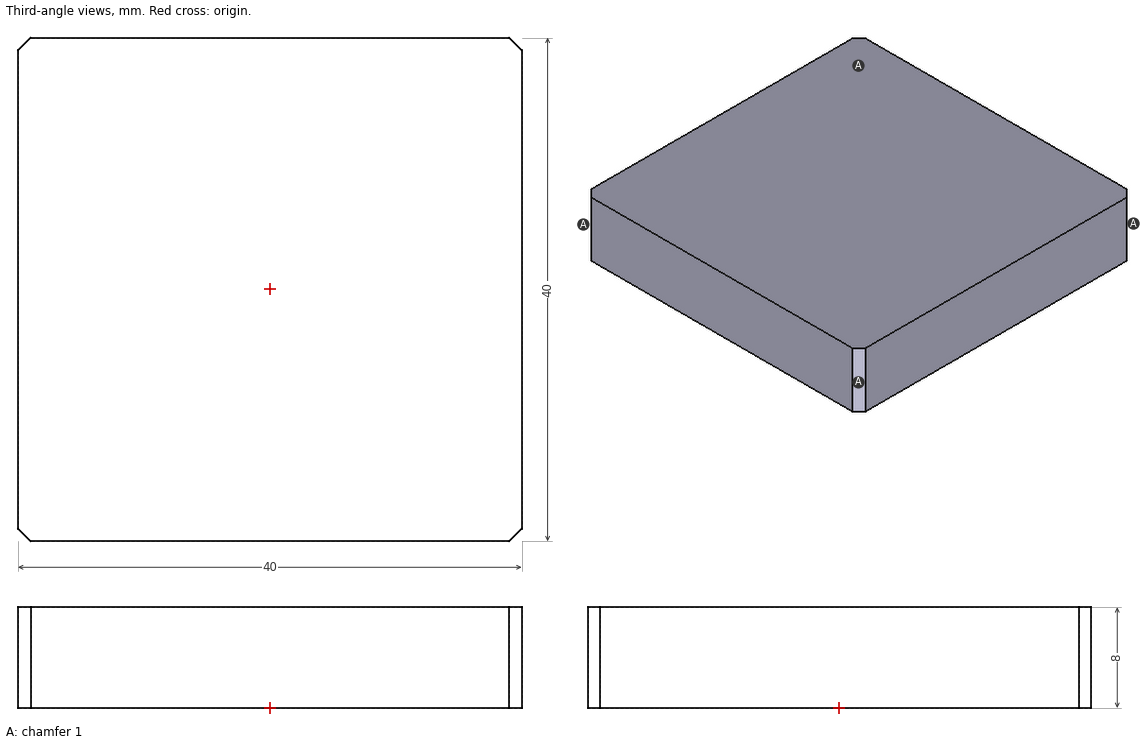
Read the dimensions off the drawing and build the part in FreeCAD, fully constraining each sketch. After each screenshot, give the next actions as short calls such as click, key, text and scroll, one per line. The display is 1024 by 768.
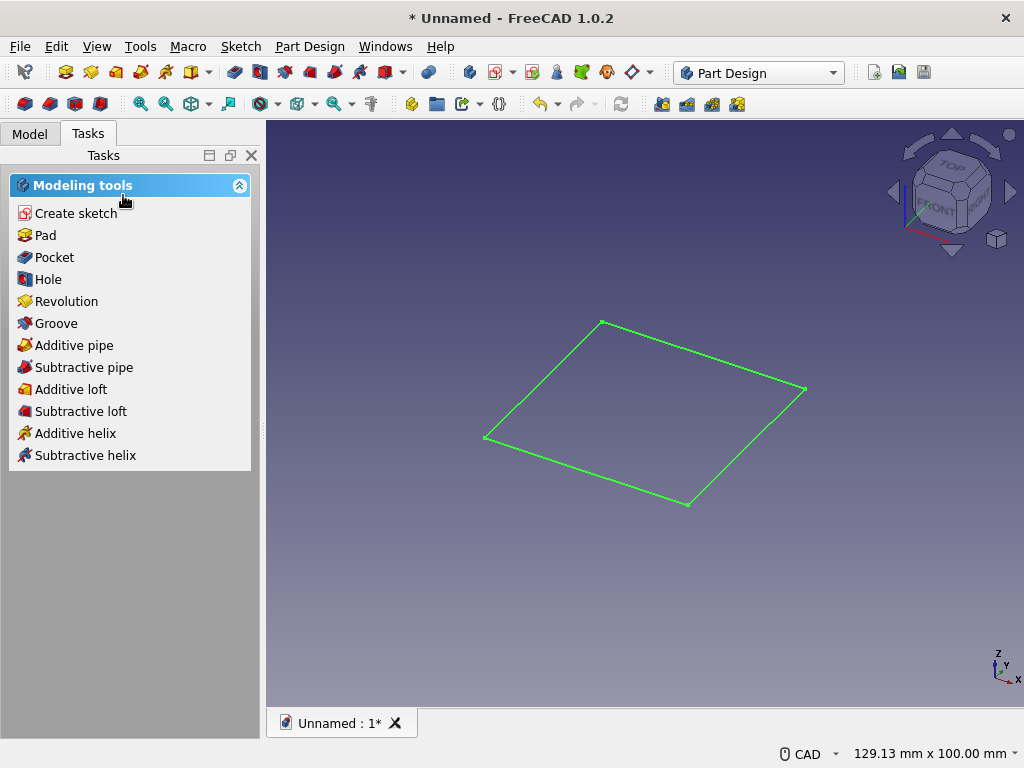
click(66, 72)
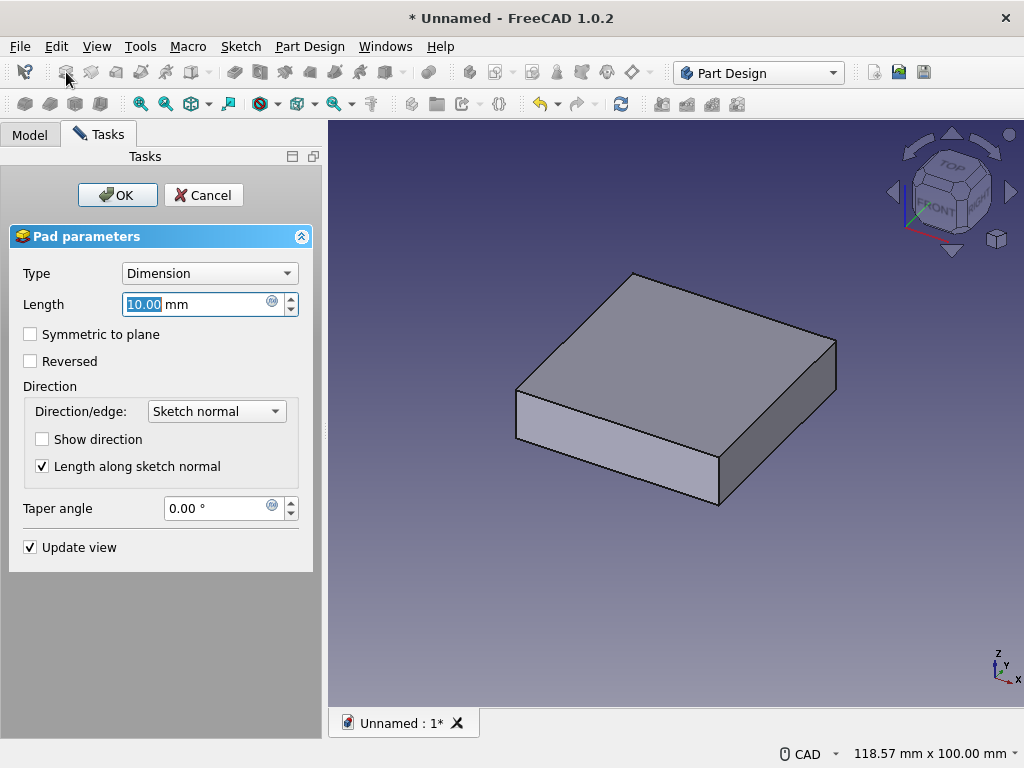
text(8)
key(Tab)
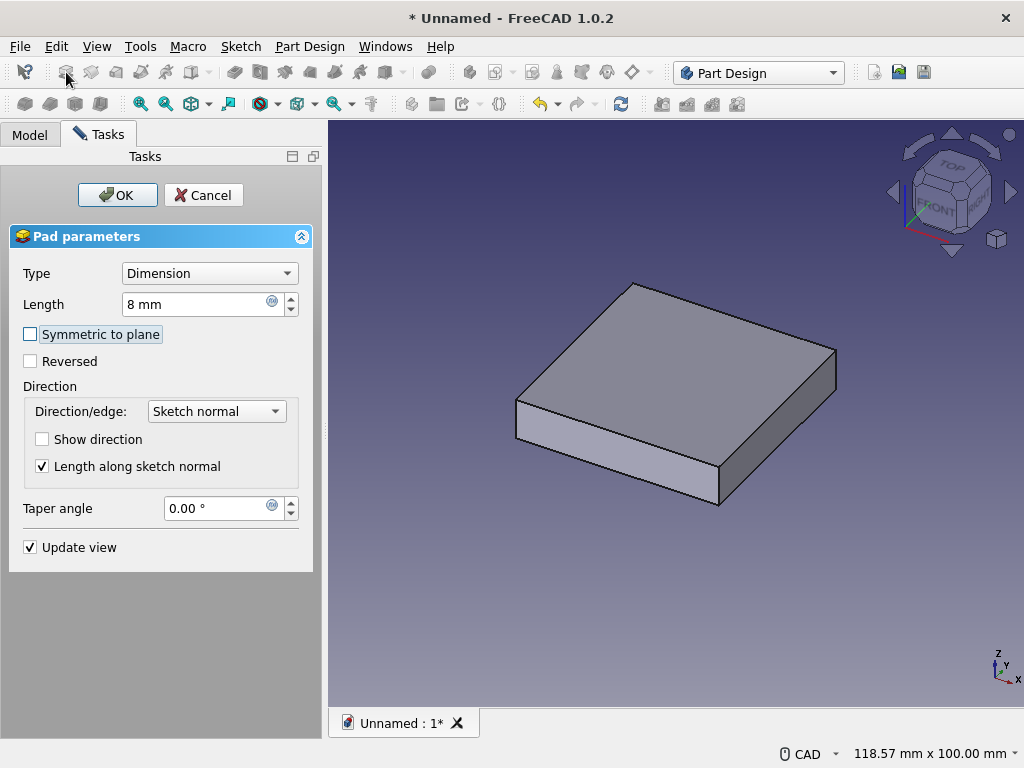
click(118, 195)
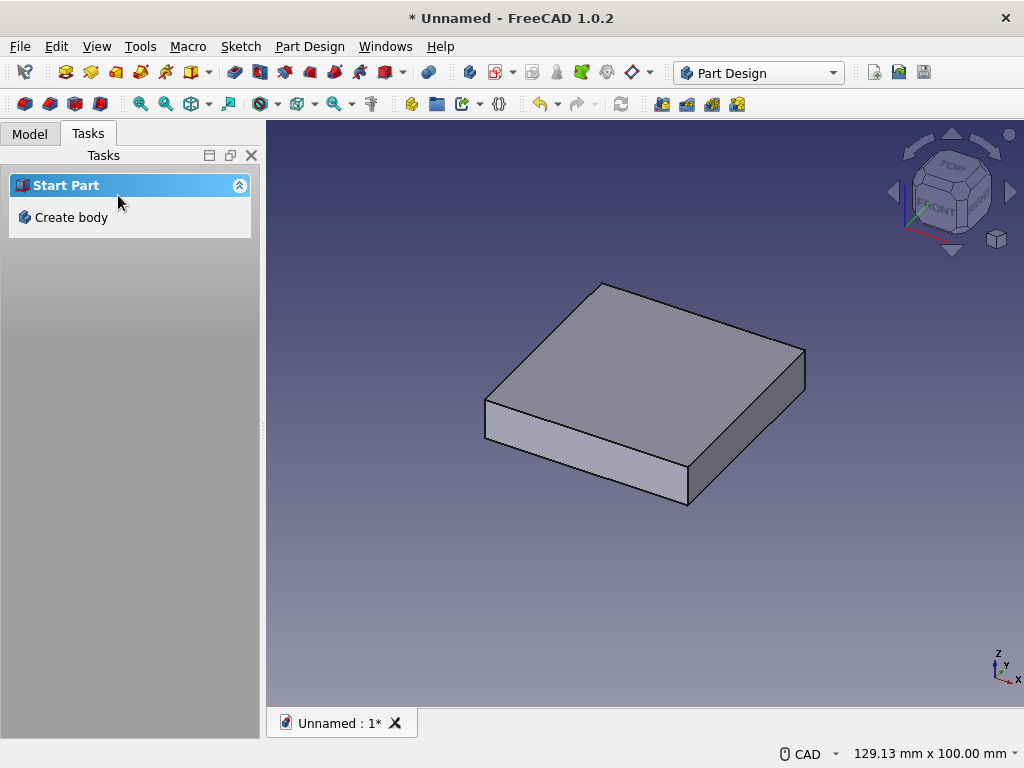
click(141, 104)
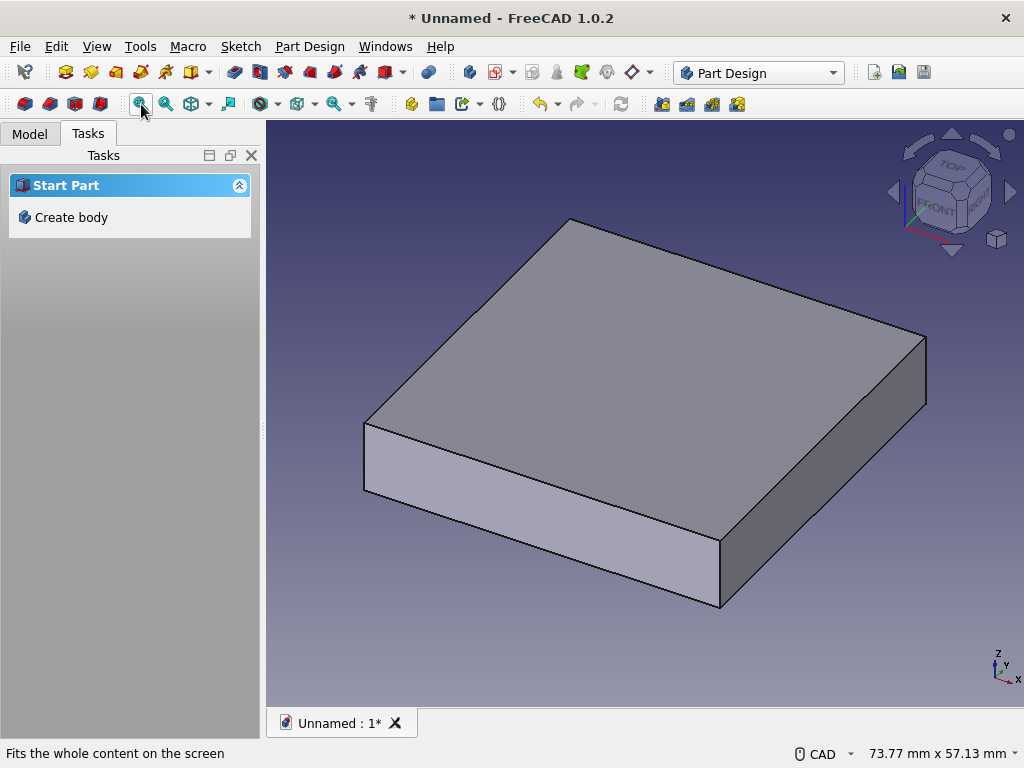
click(720, 574)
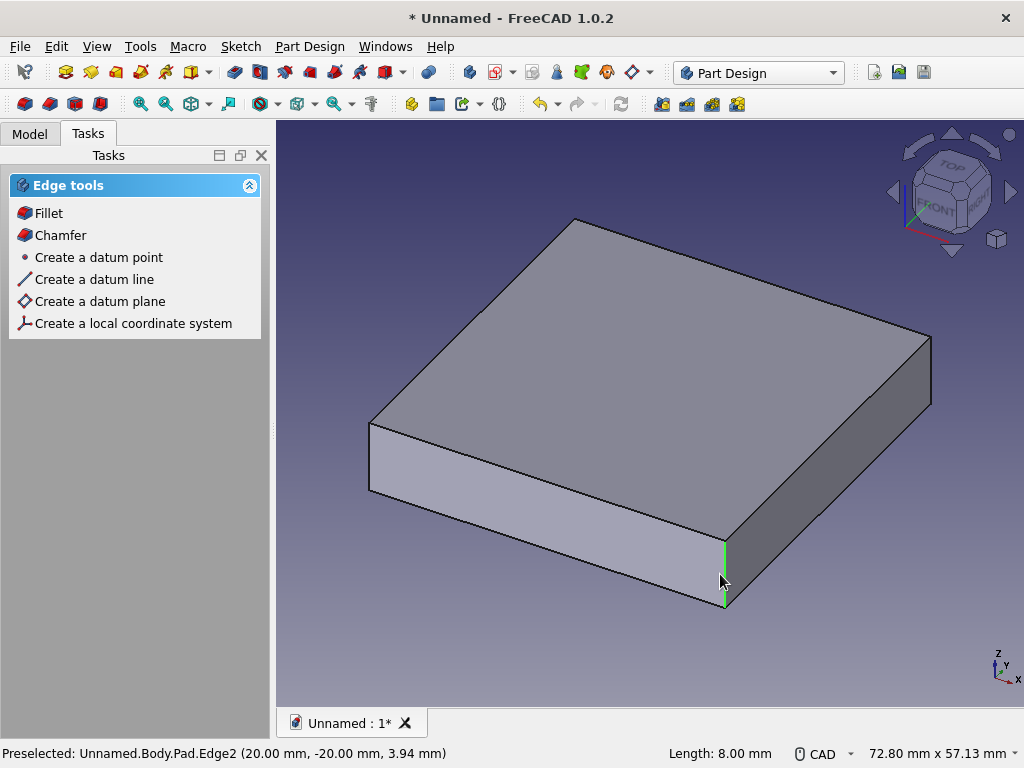
key(0)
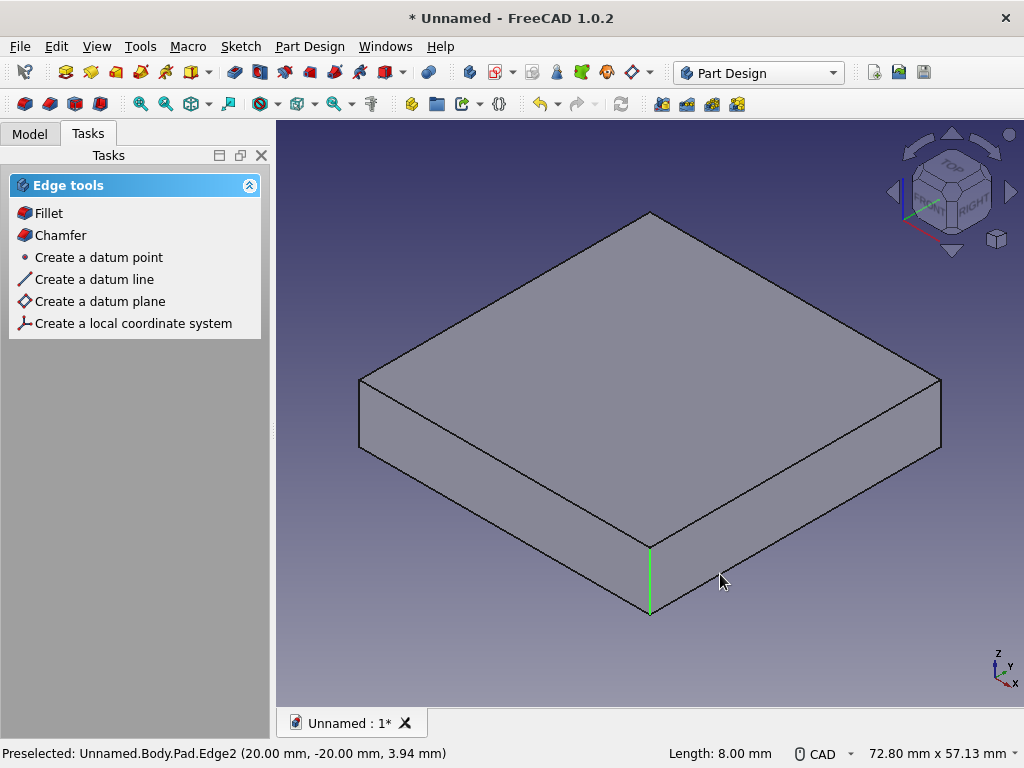
key(2)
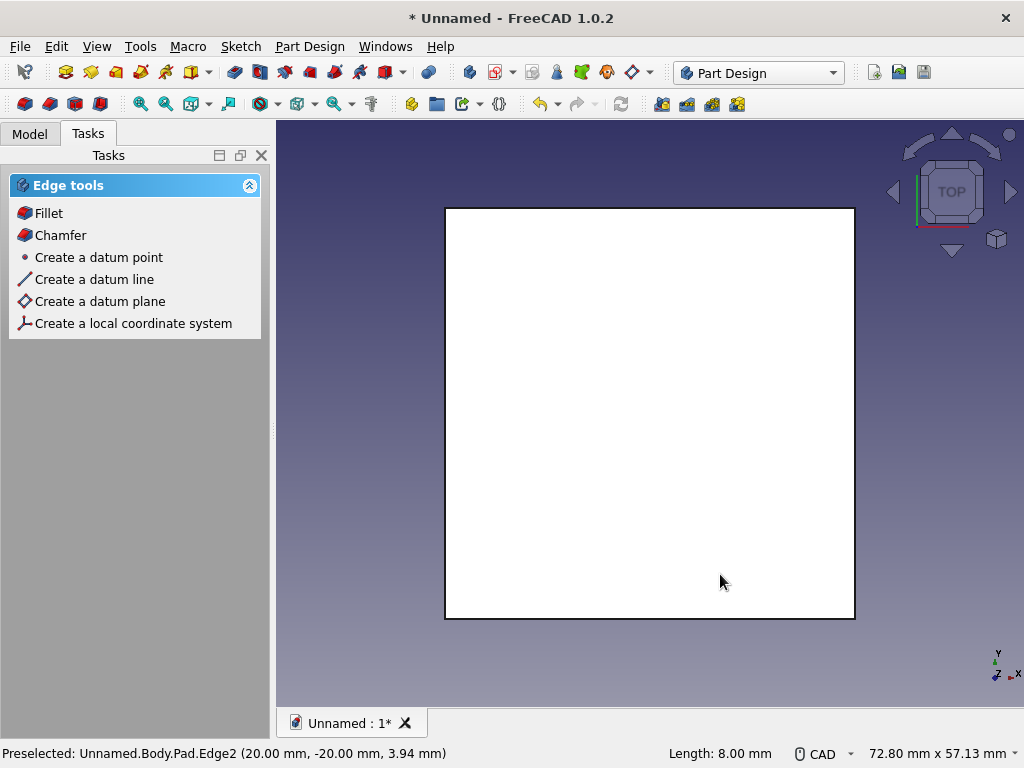
key(1)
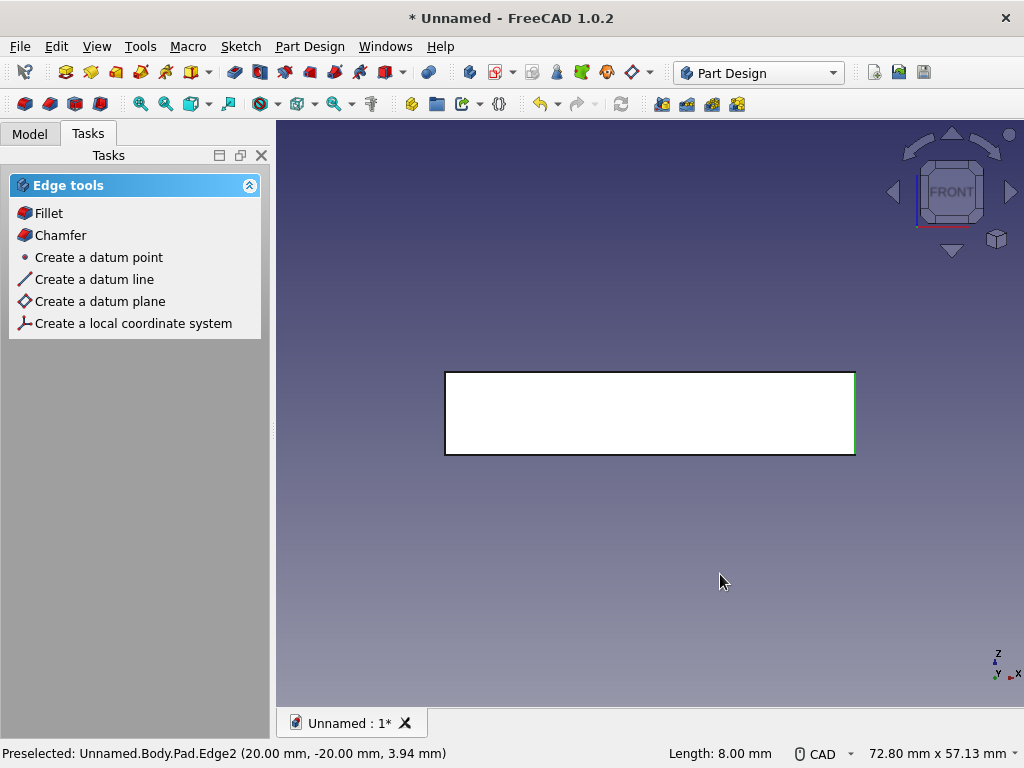
click(445, 412, ctrl)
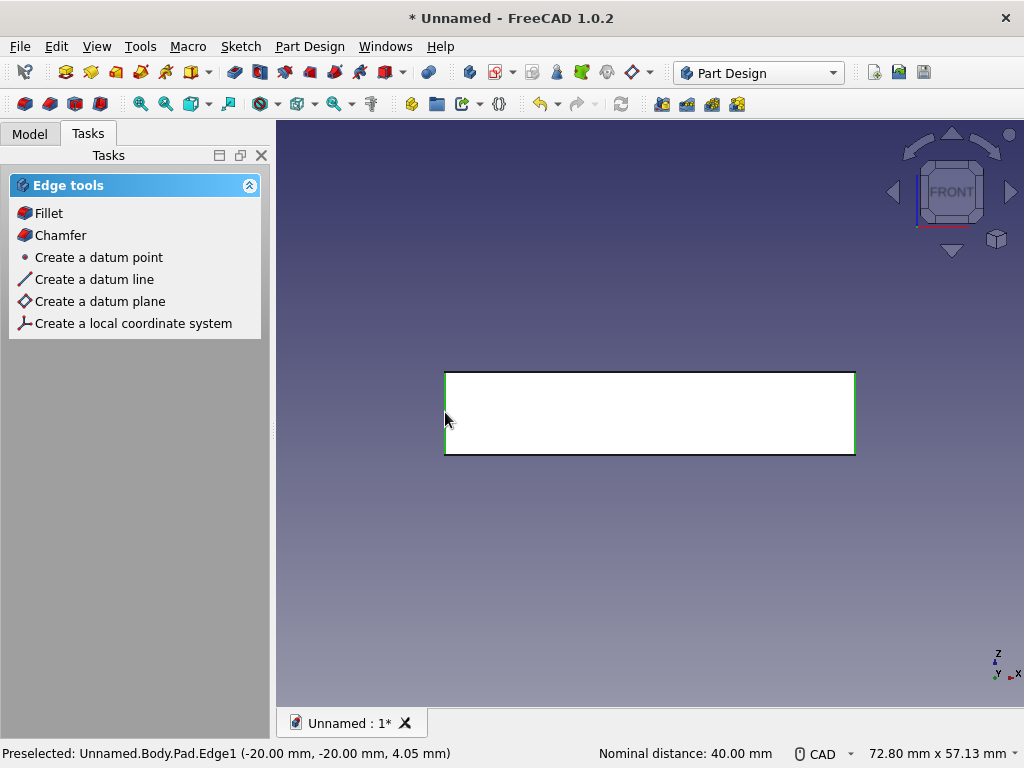
key(3)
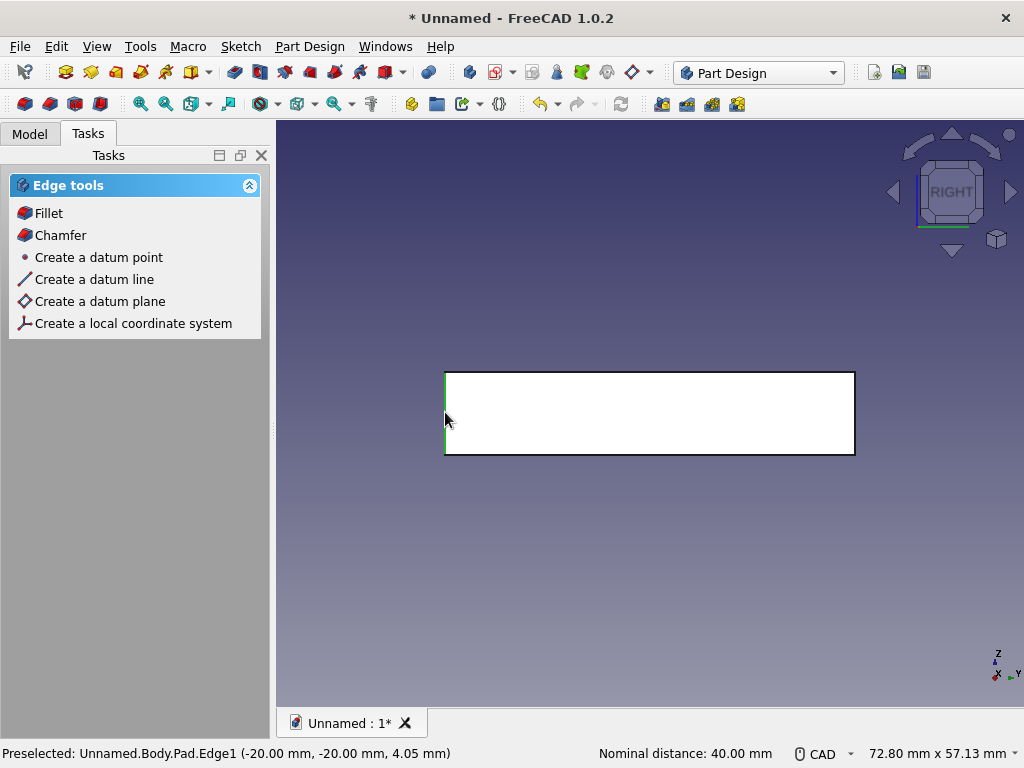
click(855, 412, ctrl)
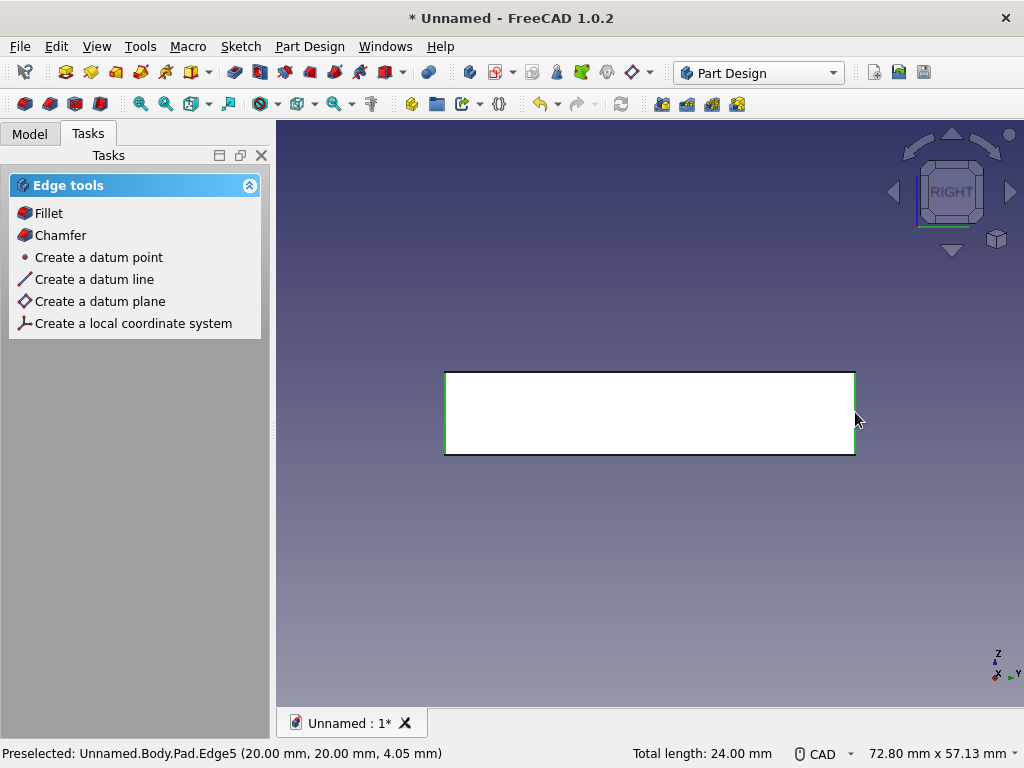
key(5)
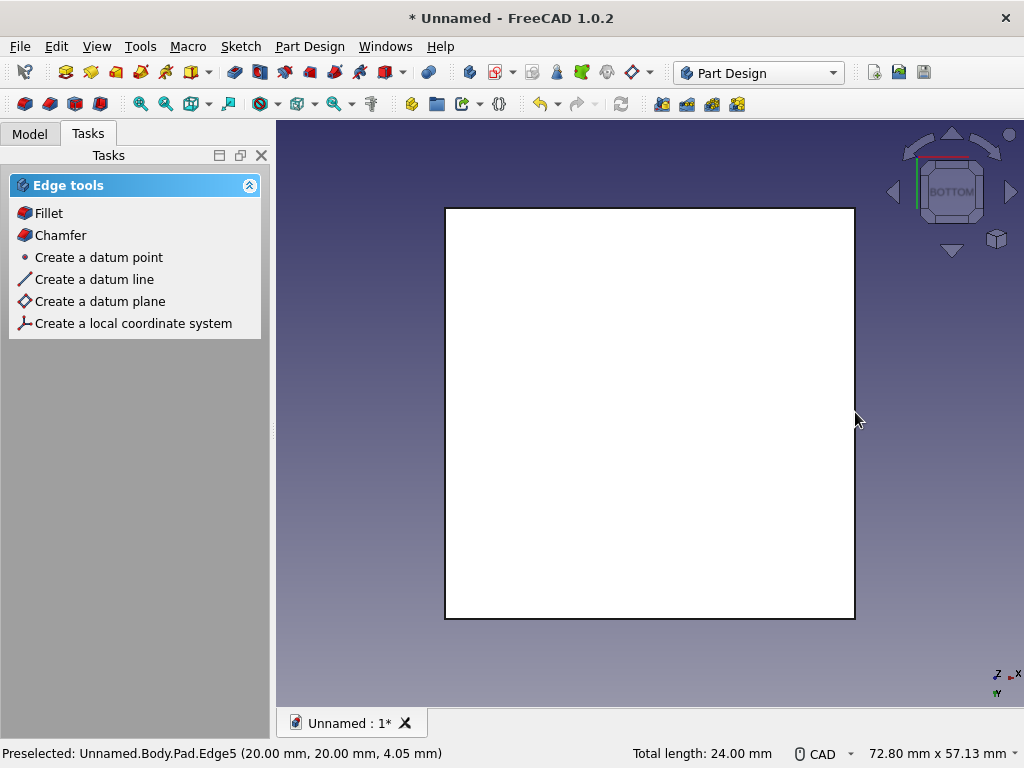
key(4)